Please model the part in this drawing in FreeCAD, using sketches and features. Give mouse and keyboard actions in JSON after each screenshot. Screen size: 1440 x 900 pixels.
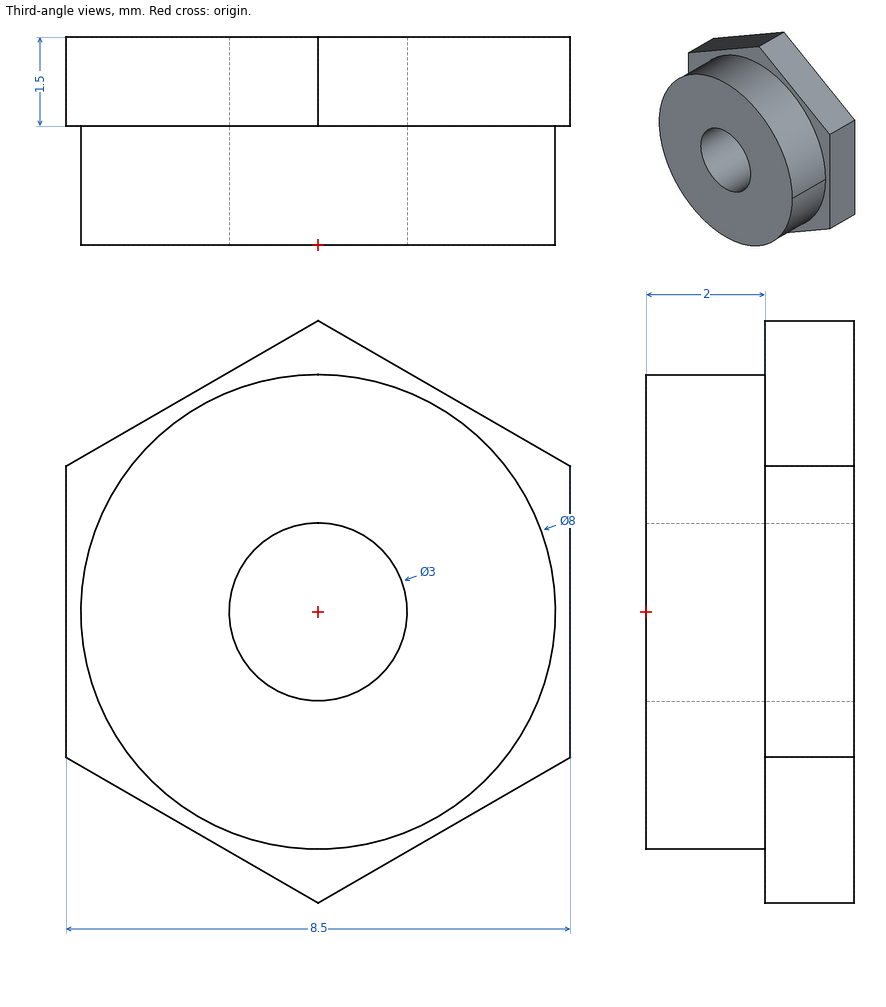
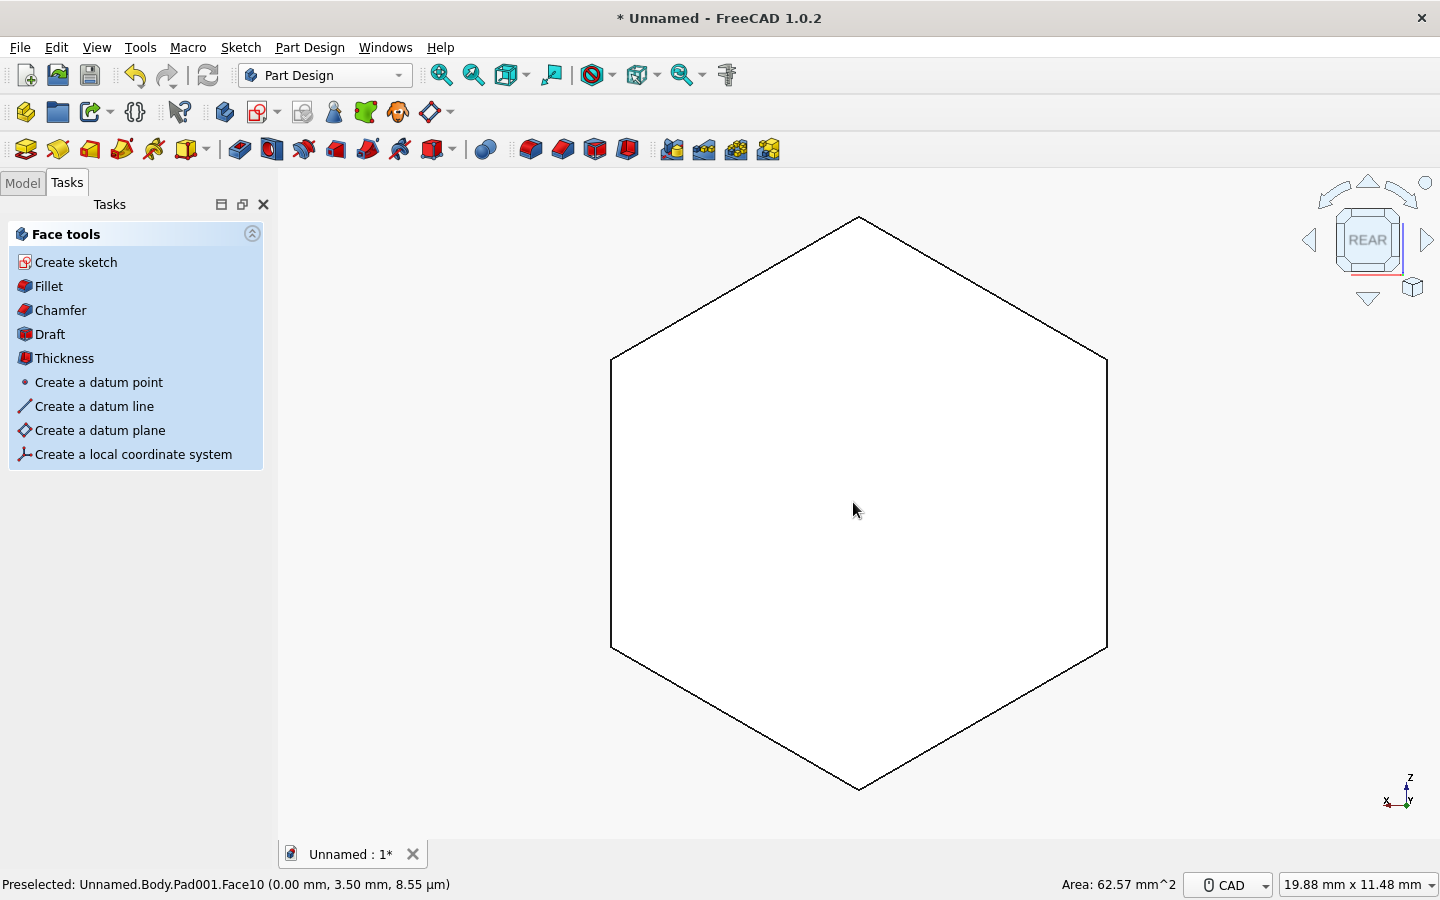
{"action": "left_click", "coordinate": [258, 112]}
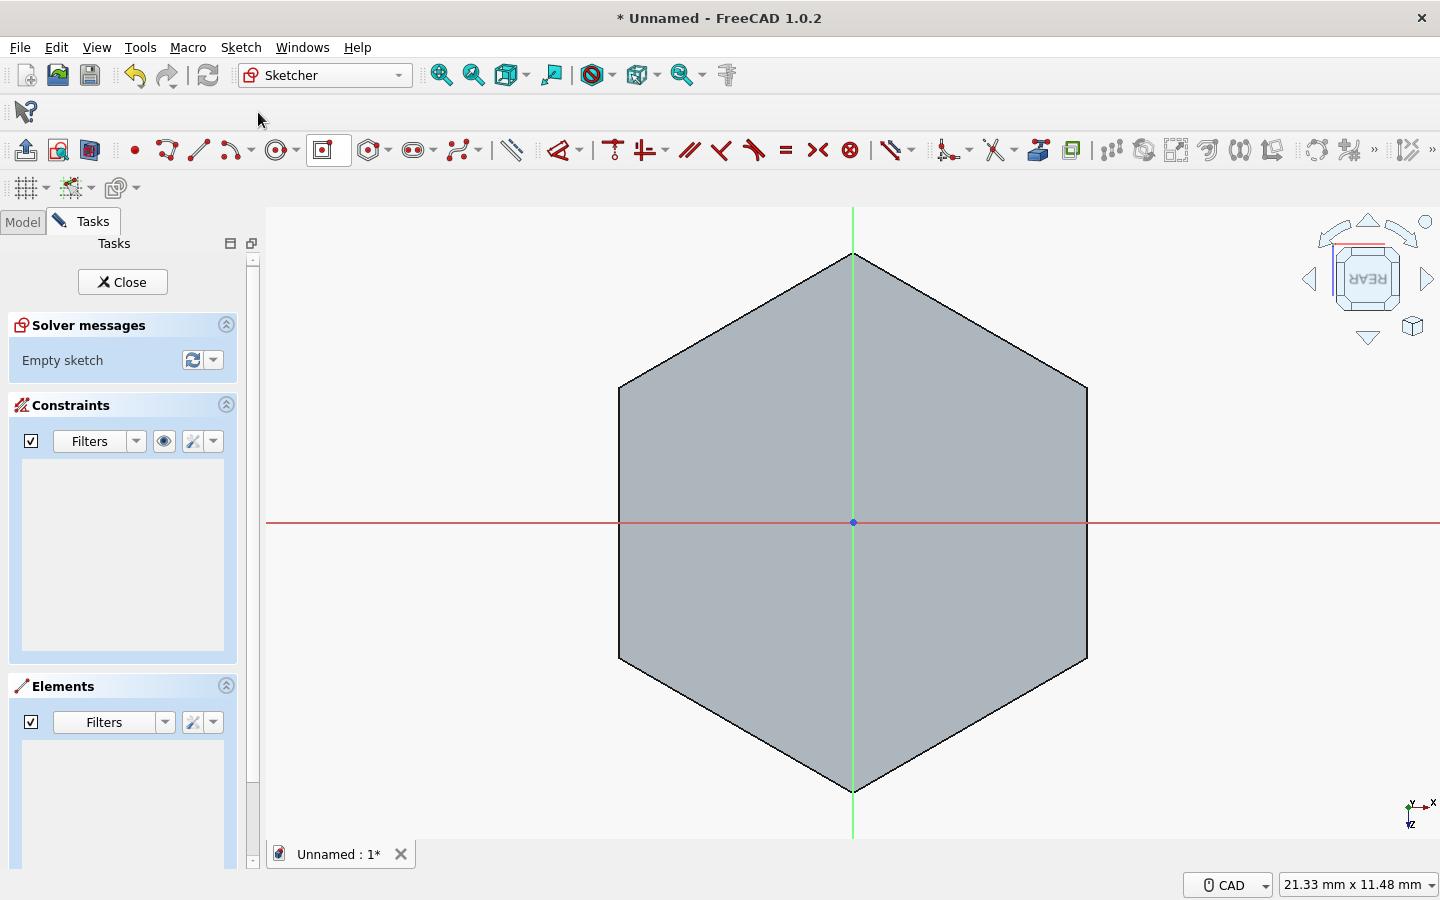
{"action": "scroll", "coordinate": [893, 523], "scroll_direction": "up", "scroll_amount": 5}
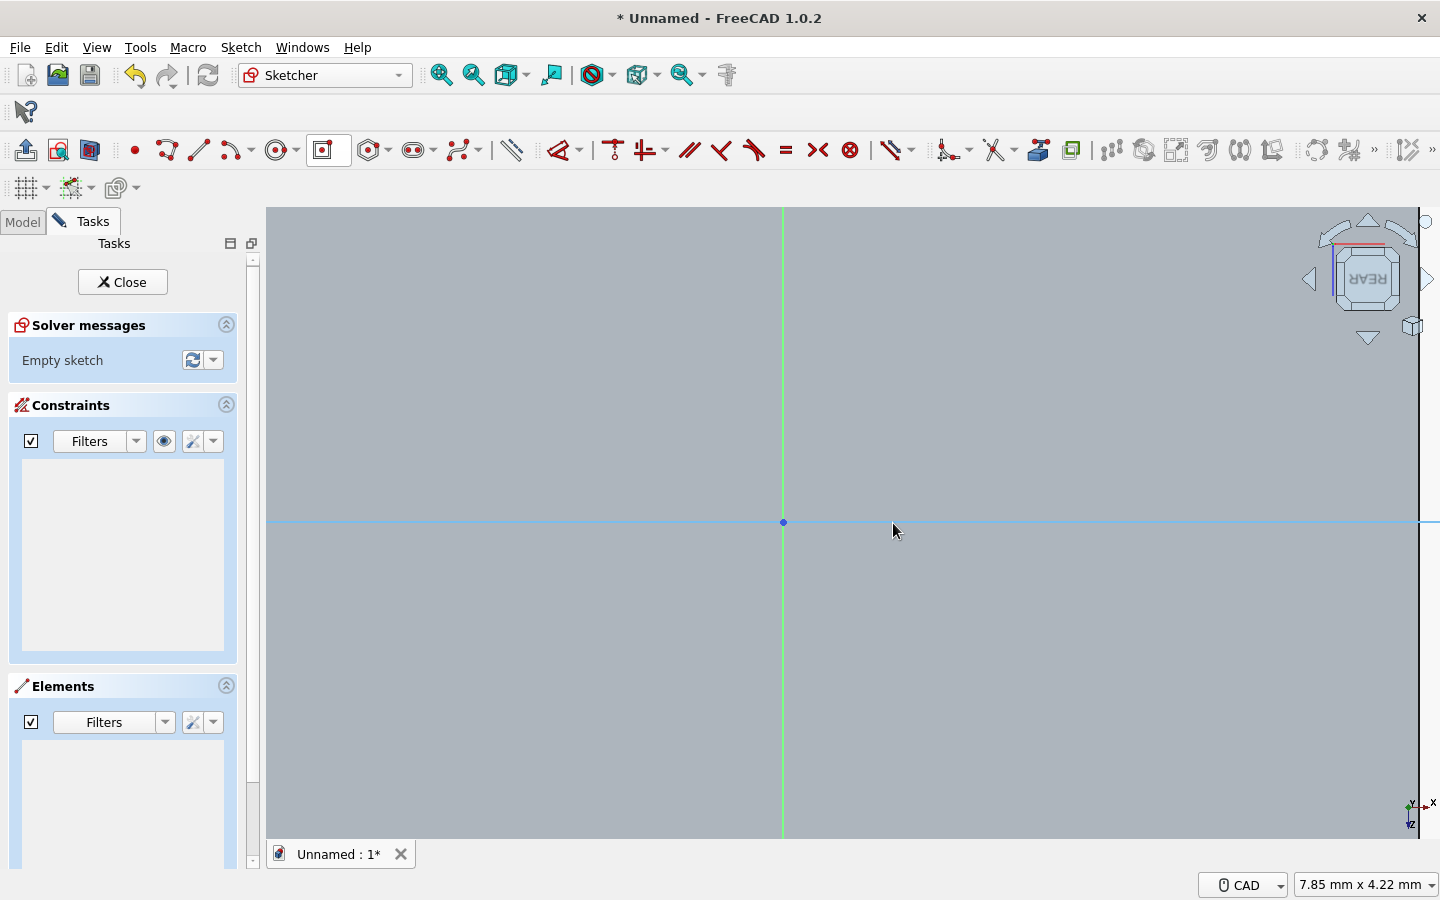
{"action": "key", "text": "g c"}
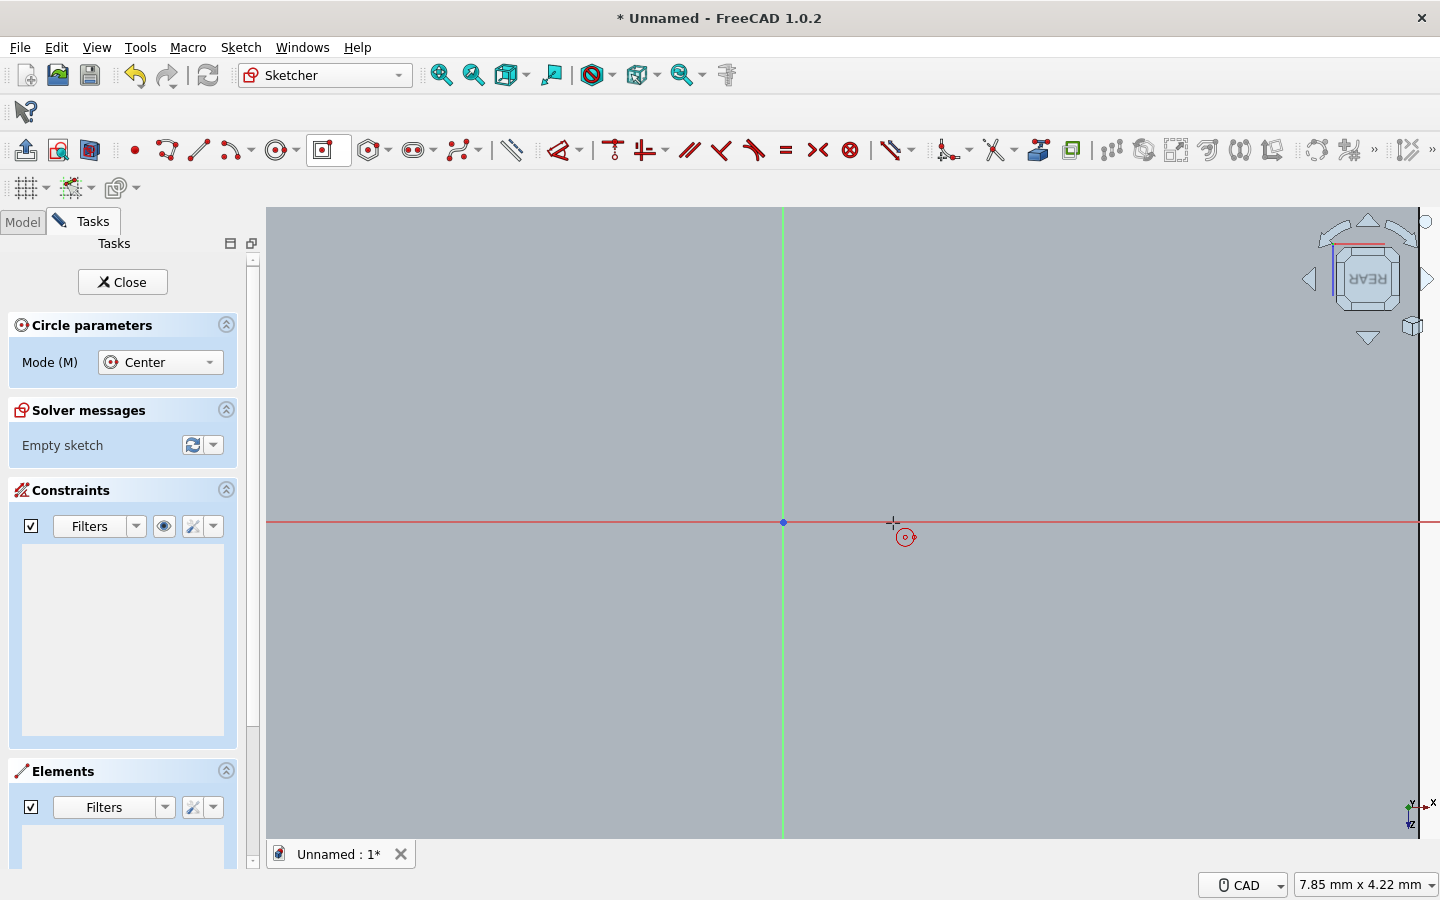
{"action": "left_click", "coordinate": [783, 522]}
{"action": "mouse_move", "coordinate": [942, 363]}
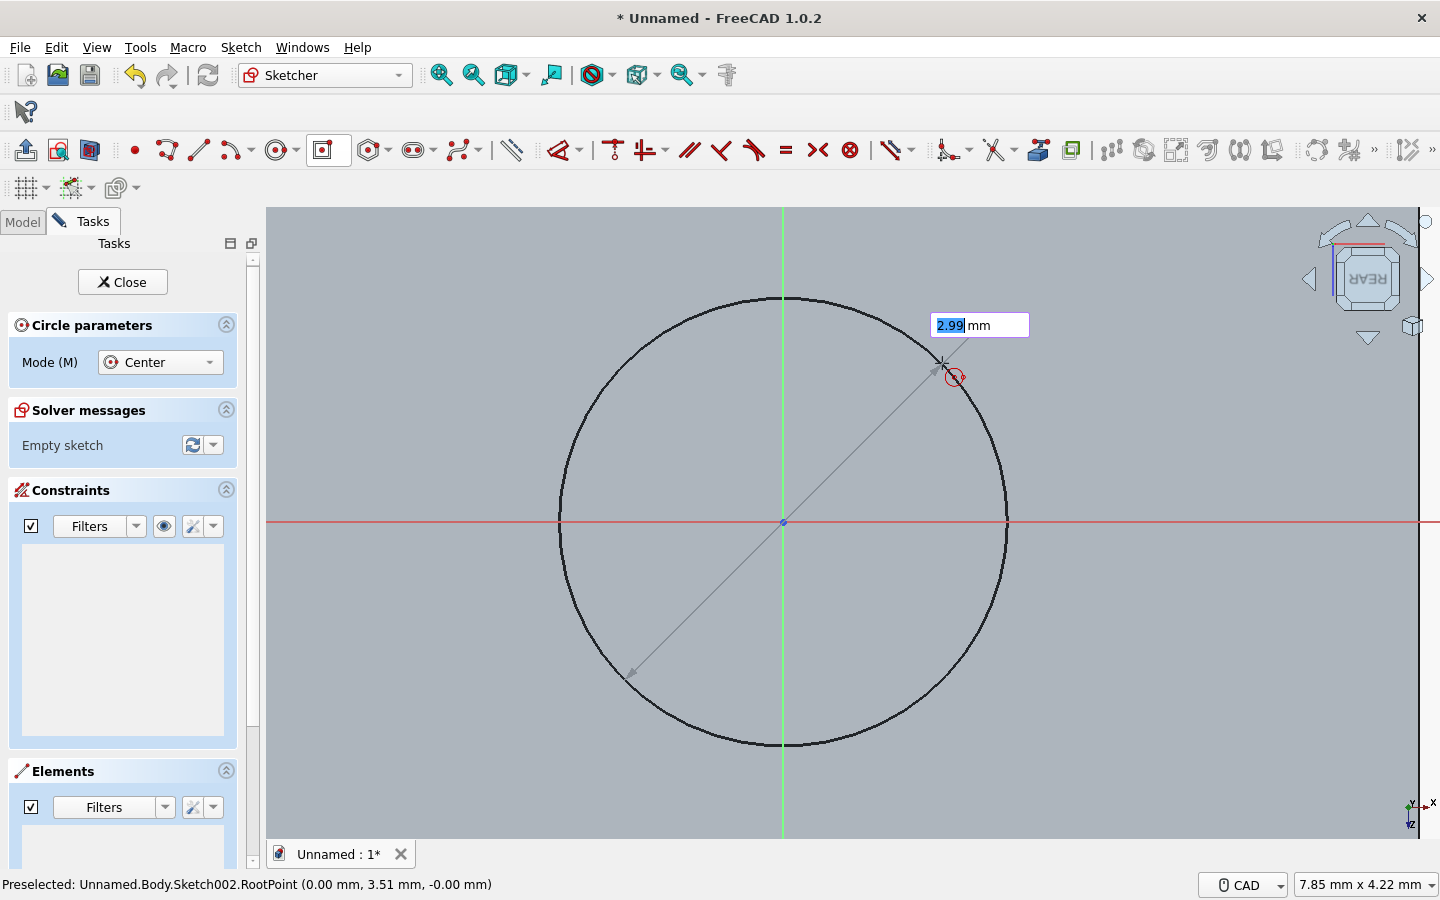
{"action": "type", "text": "3"}
{"action": "key", "text": "Return"}
{"action": "key", "text": "Escape"}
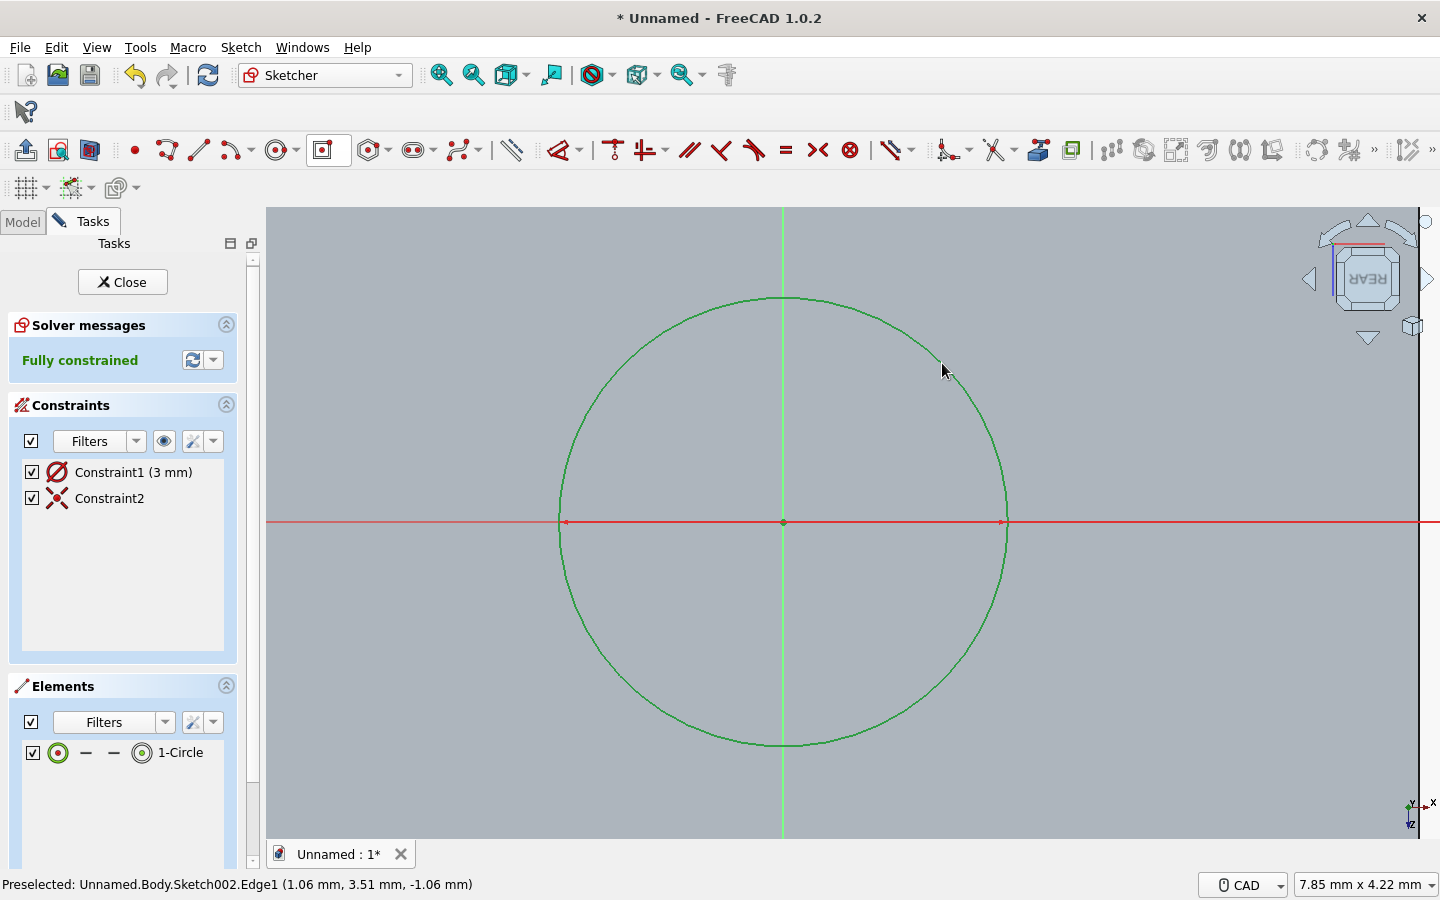
{"action": "left_click", "coordinate": [123, 282]}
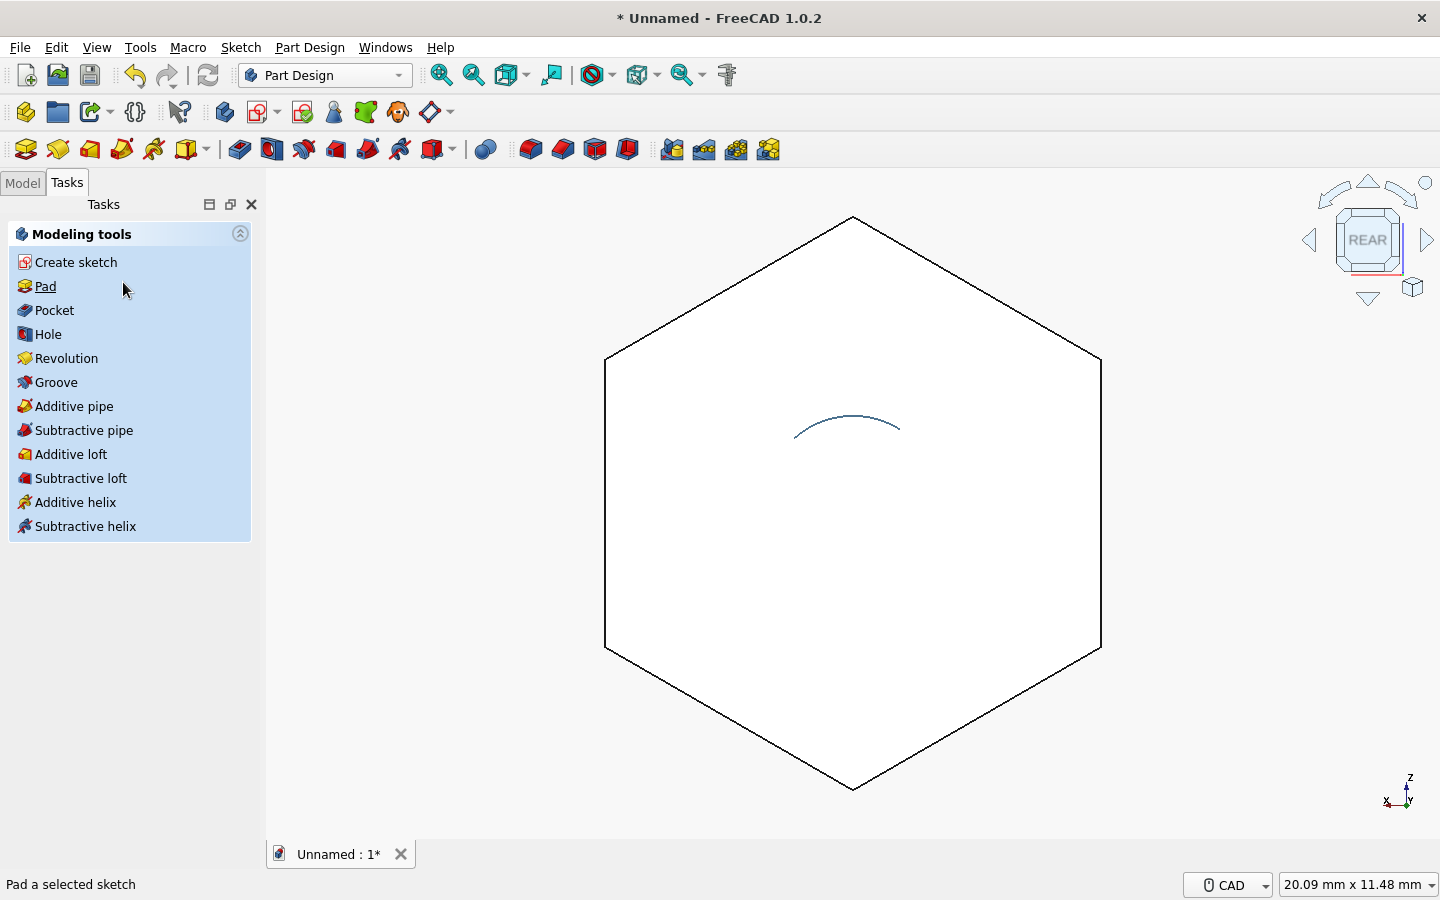
{"action": "left_click", "coordinate": [240, 150]}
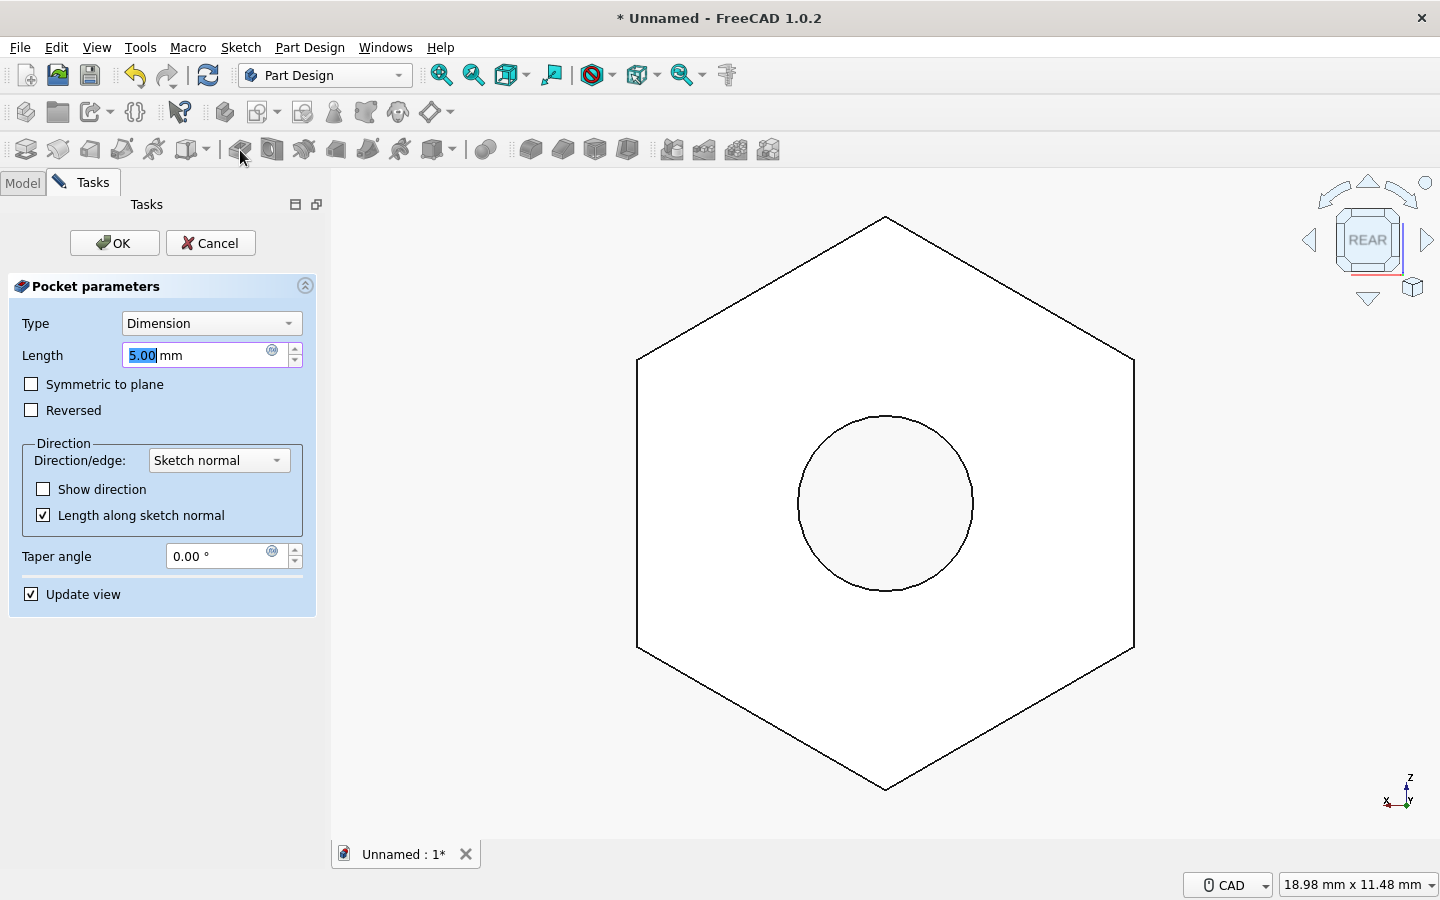
{"action": "left_click", "coordinate": [212, 324]}